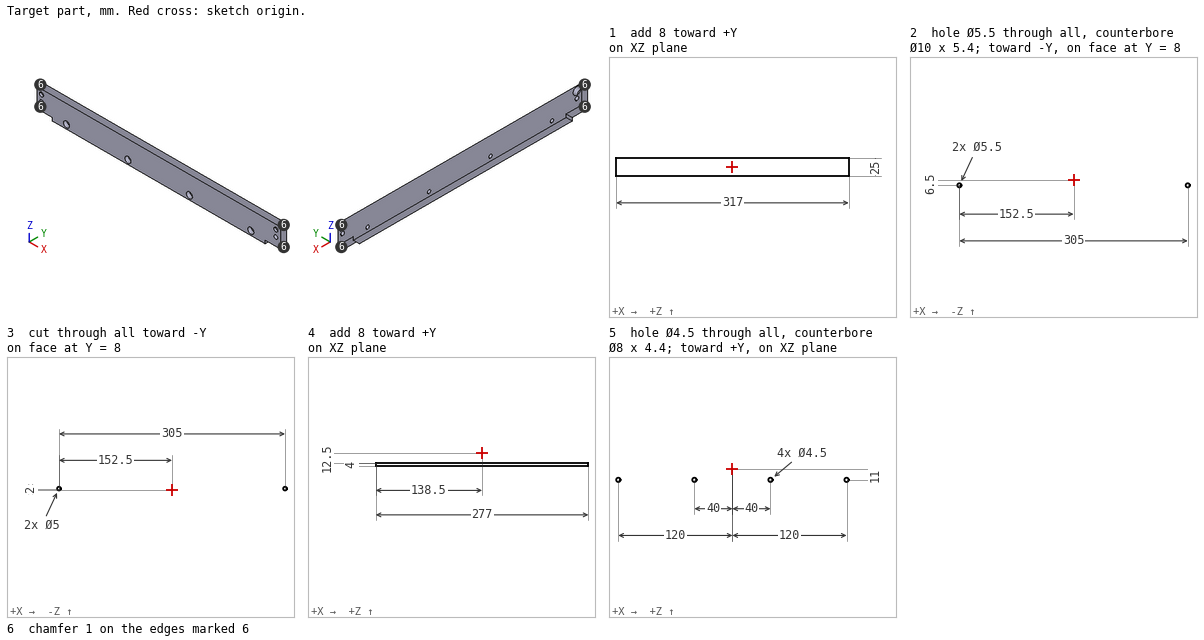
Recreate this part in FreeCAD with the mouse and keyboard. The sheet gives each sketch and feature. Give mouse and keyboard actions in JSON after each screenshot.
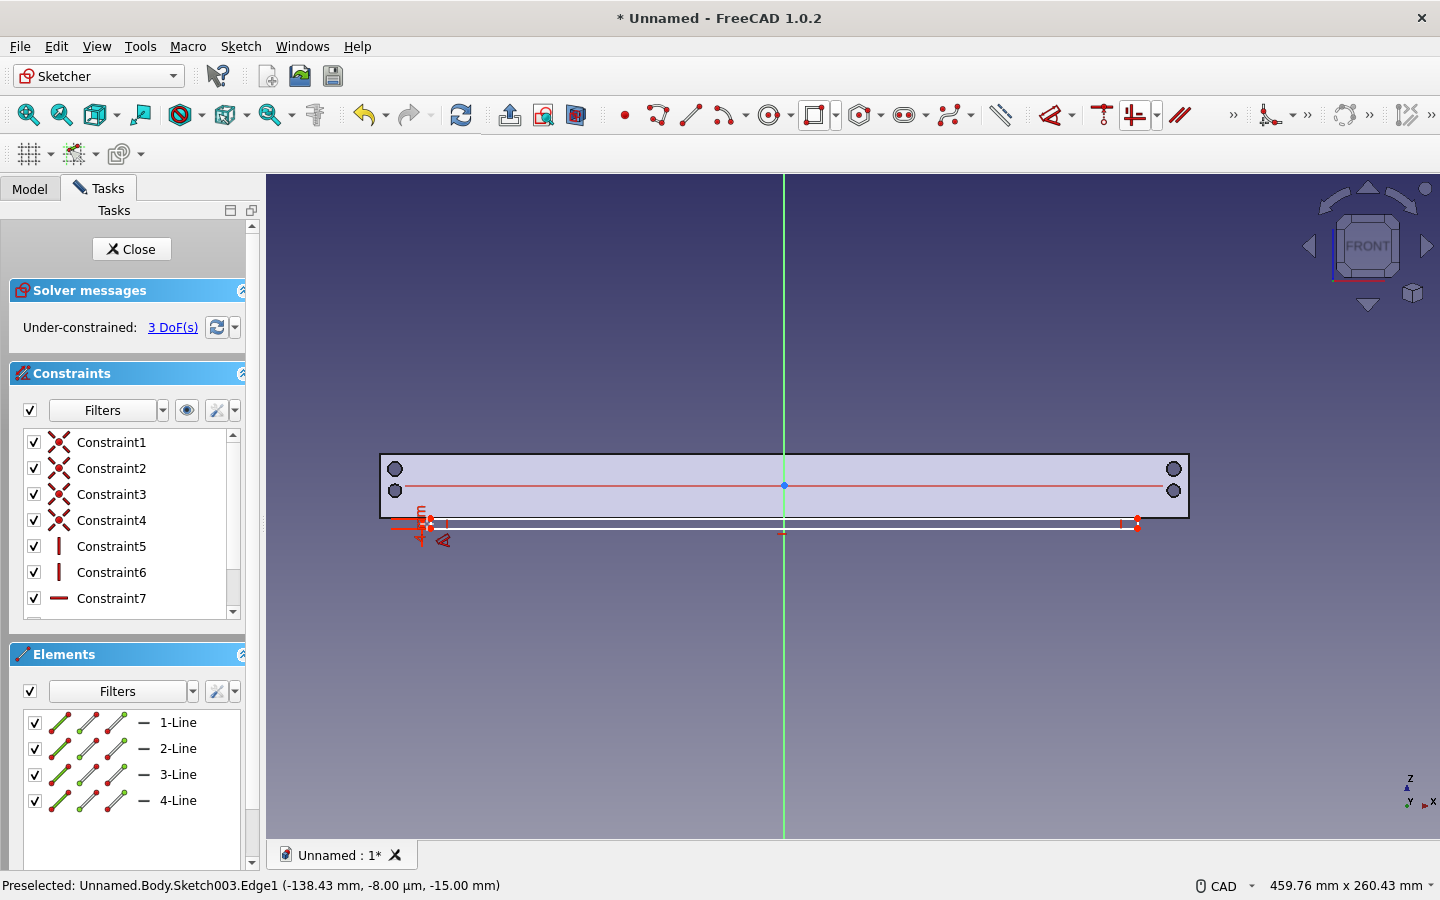
{"action": "scroll", "coordinate": [572, 529], "scroll_direction": "up", "scroll_amount": 2}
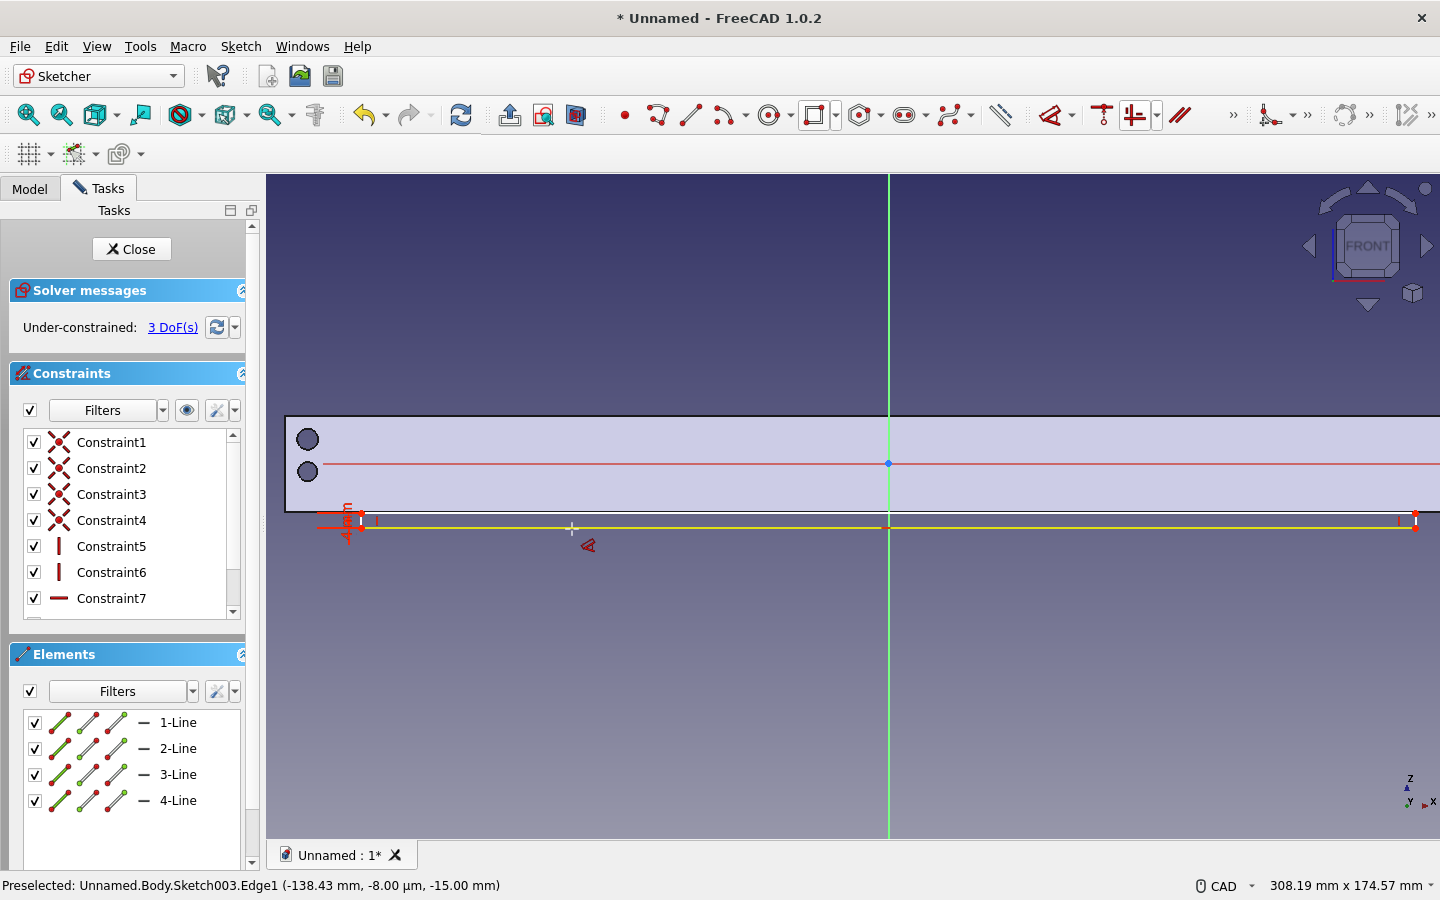
{"action": "left_click", "coordinate": [572, 528]}
{"action": "left_click", "coordinate": [818, 562]}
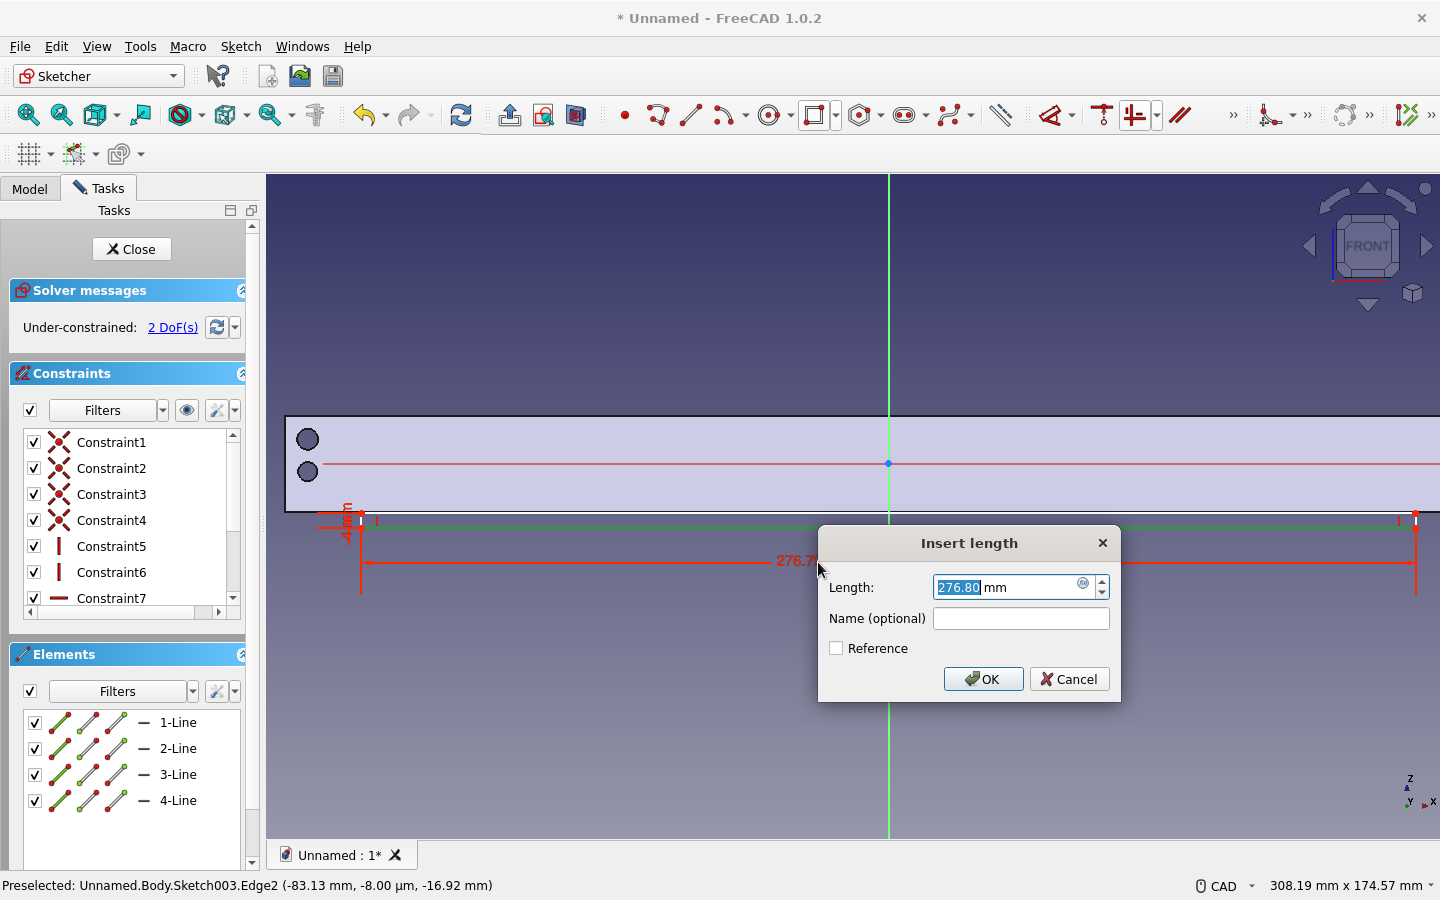
{"action": "type", "text": "277"}
{"action": "key", "text": "Return"}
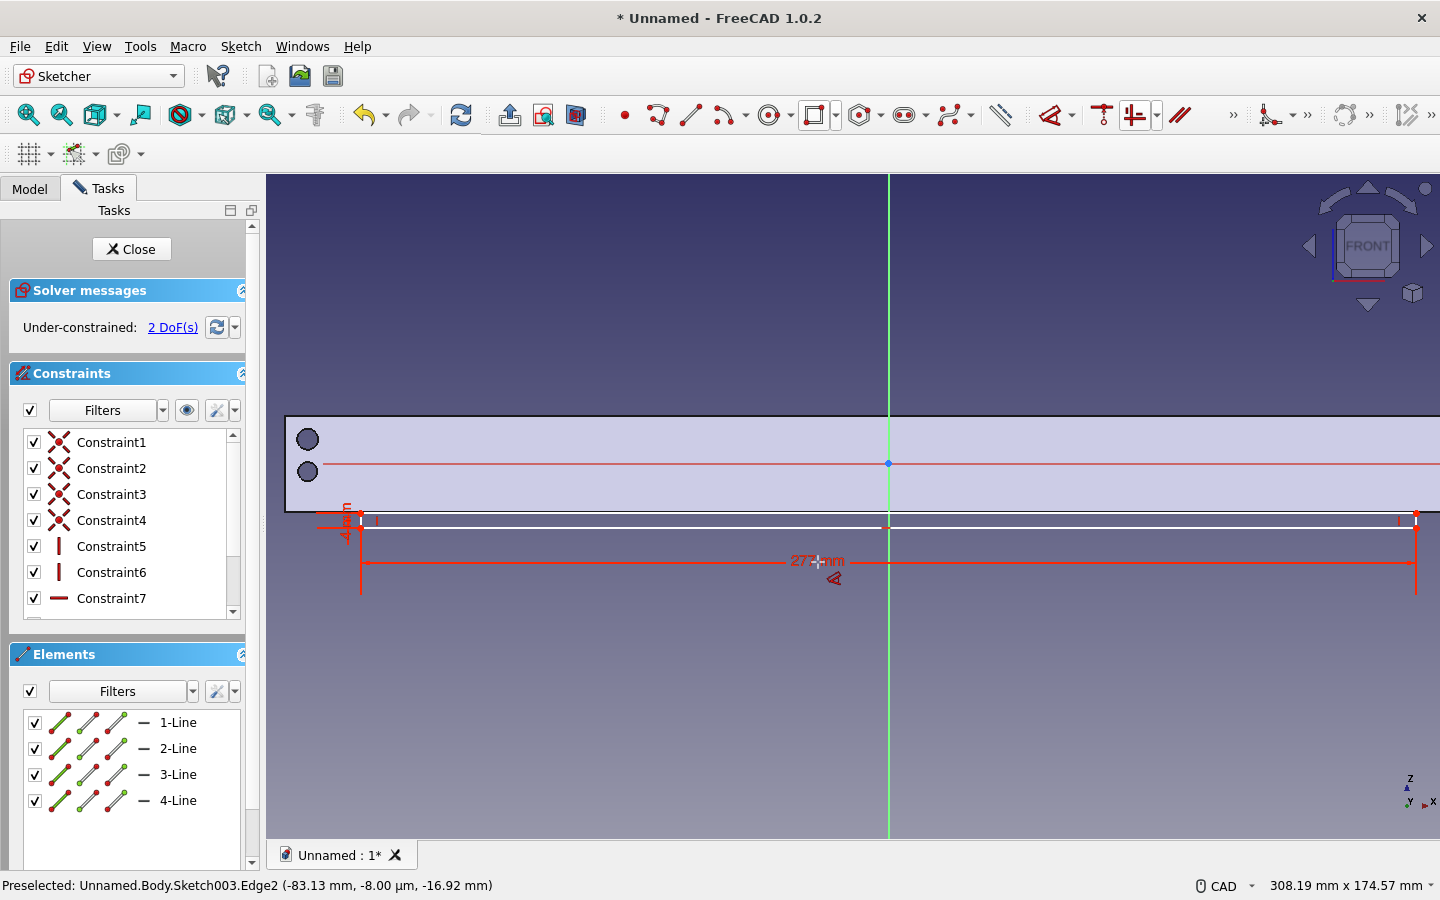
{"action": "left_click", "coordinate": [361, 513]}
{"action": "left_click", "coordinate": [327, 489]}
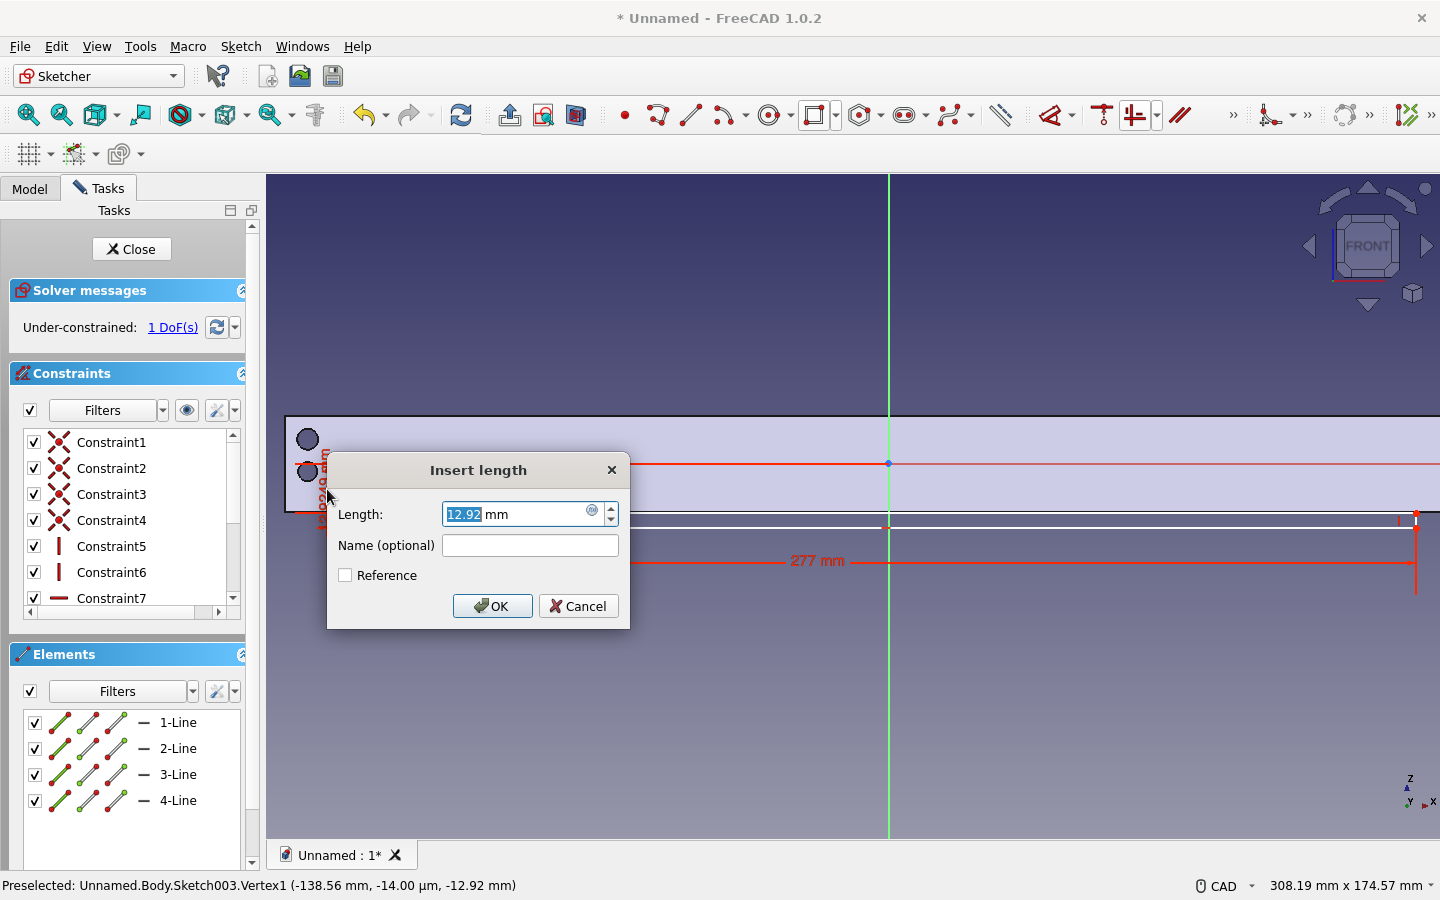
{"action": "type", "text": "12.5"}
{"action": "key", "text": "Return"}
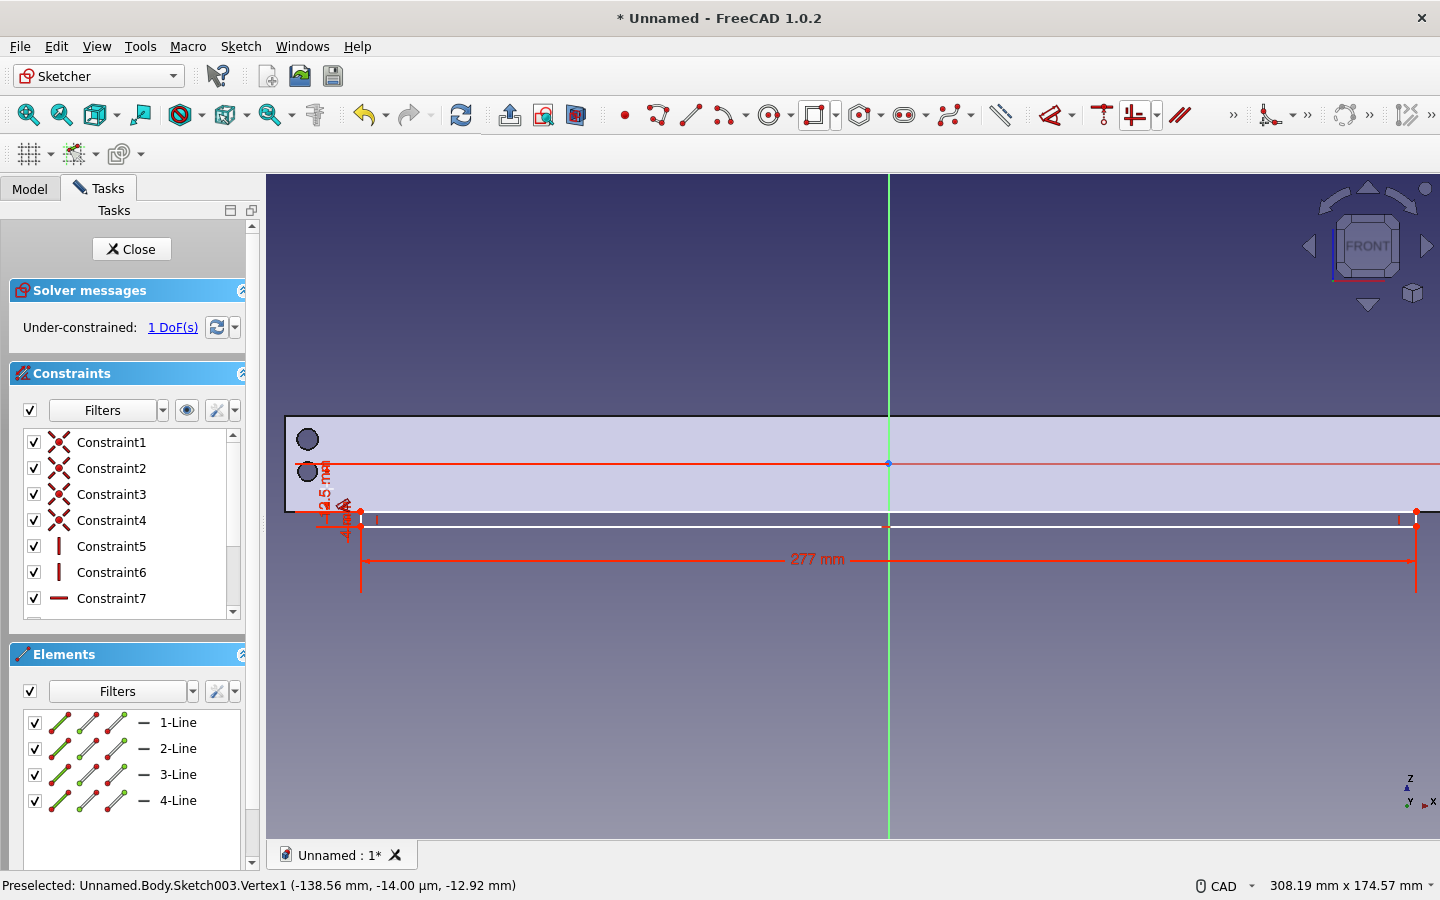
{"action": "left_click", "coordinate": [361, 512]}
{"action": "left_click", "coordinate": [625, 430]}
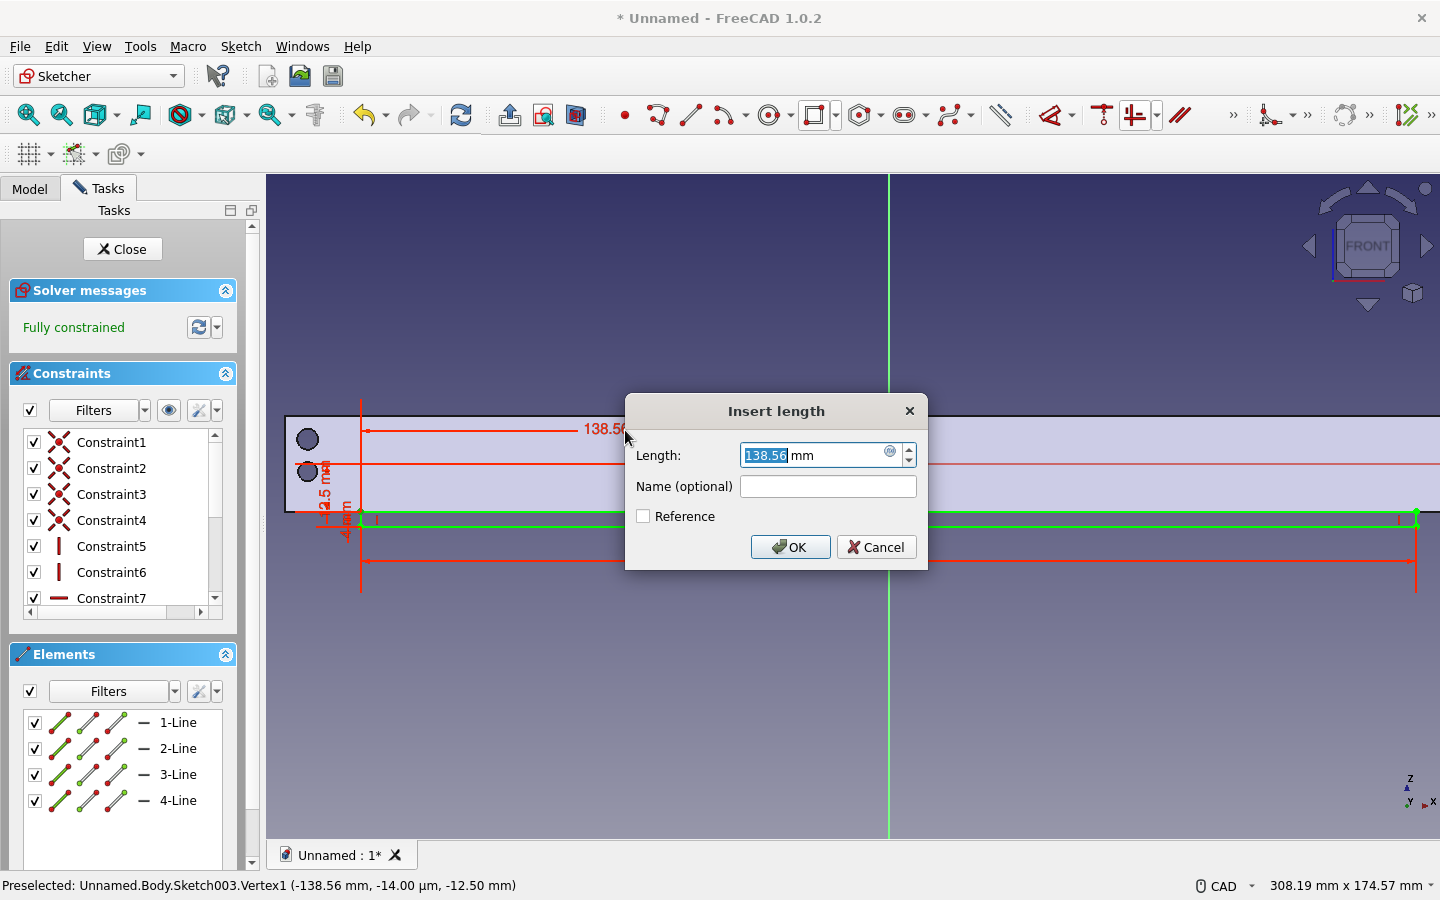
{"action": "type", "text": "138.5"}
{"action": "key", "text": "Return"}
{"action": "key", "text": "Escape"}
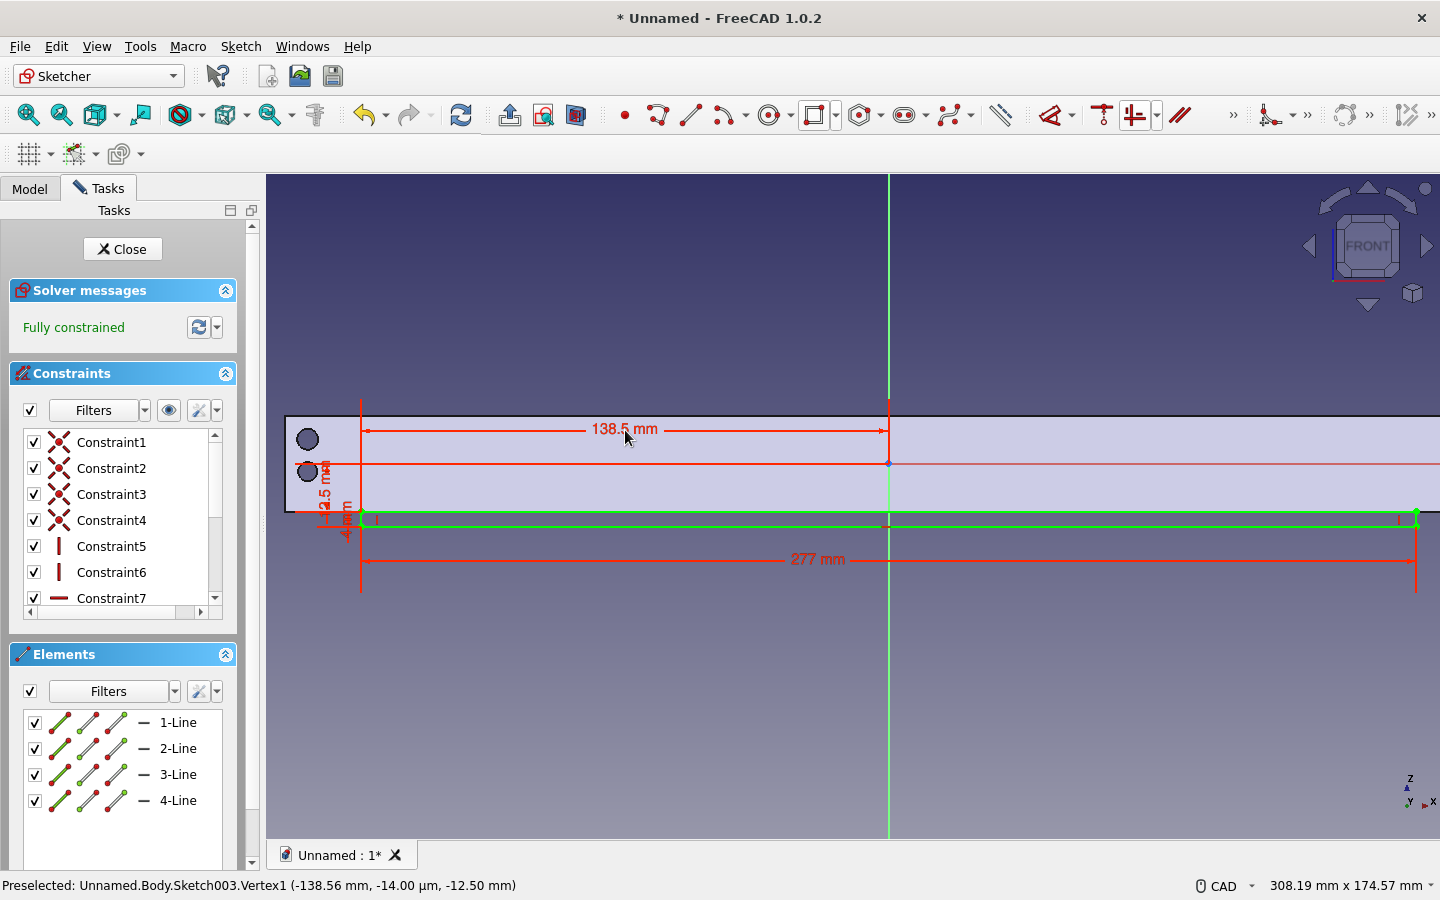
{"action": "left_click", "coordinate": [123, 249]}